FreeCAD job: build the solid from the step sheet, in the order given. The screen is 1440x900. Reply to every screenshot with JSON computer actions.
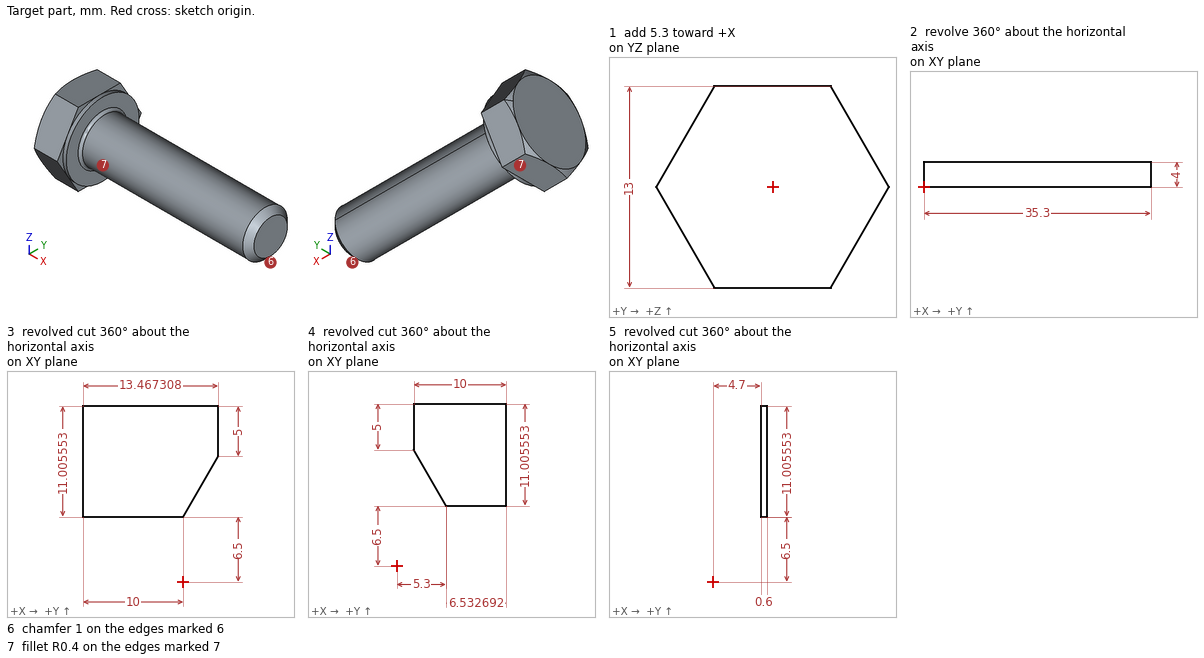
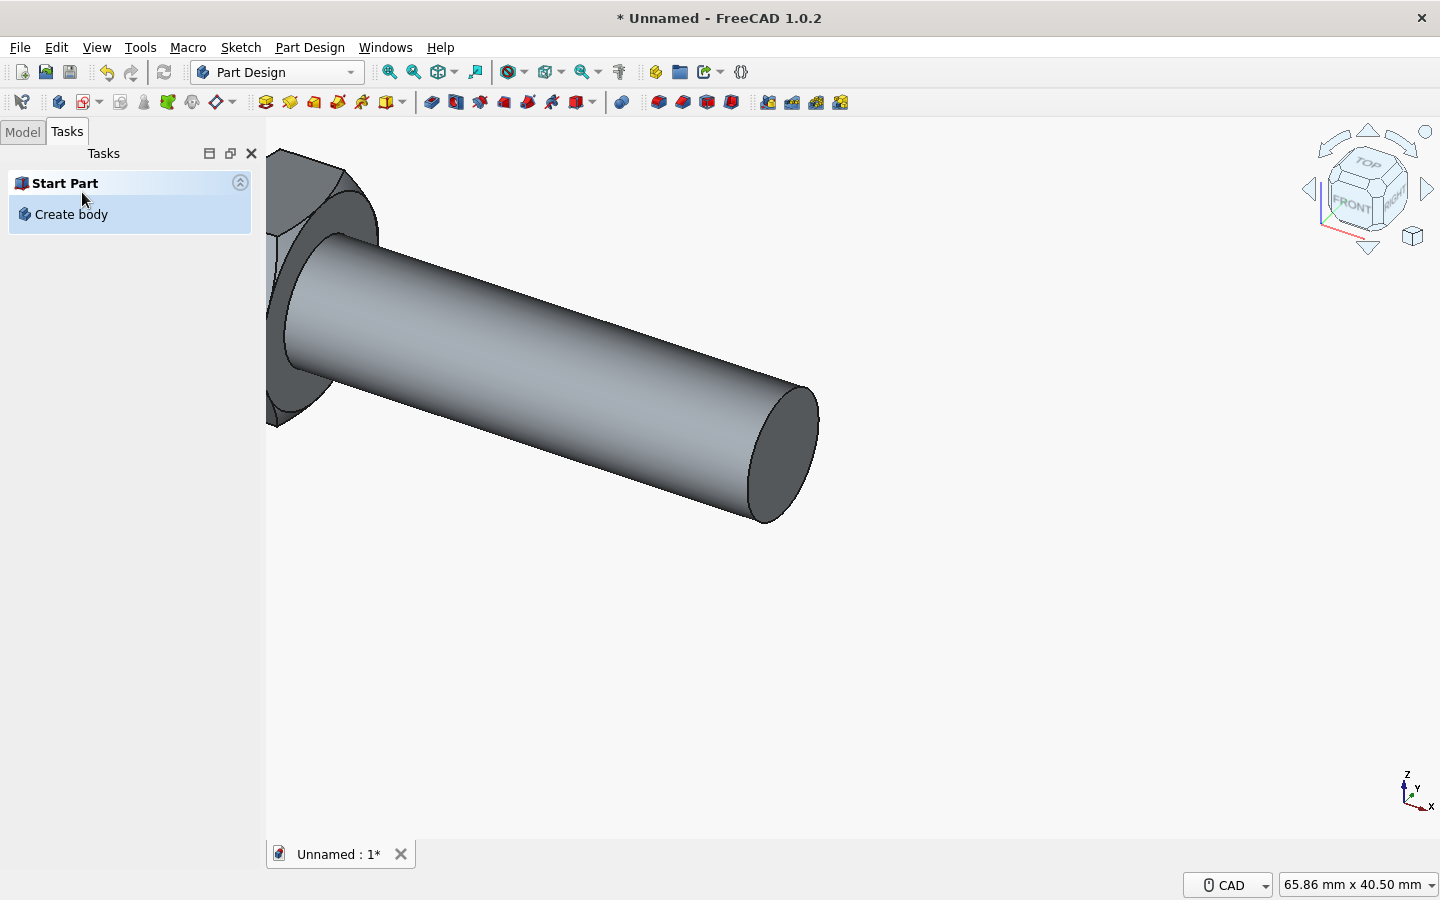
{"action": "key", "text": "v f"}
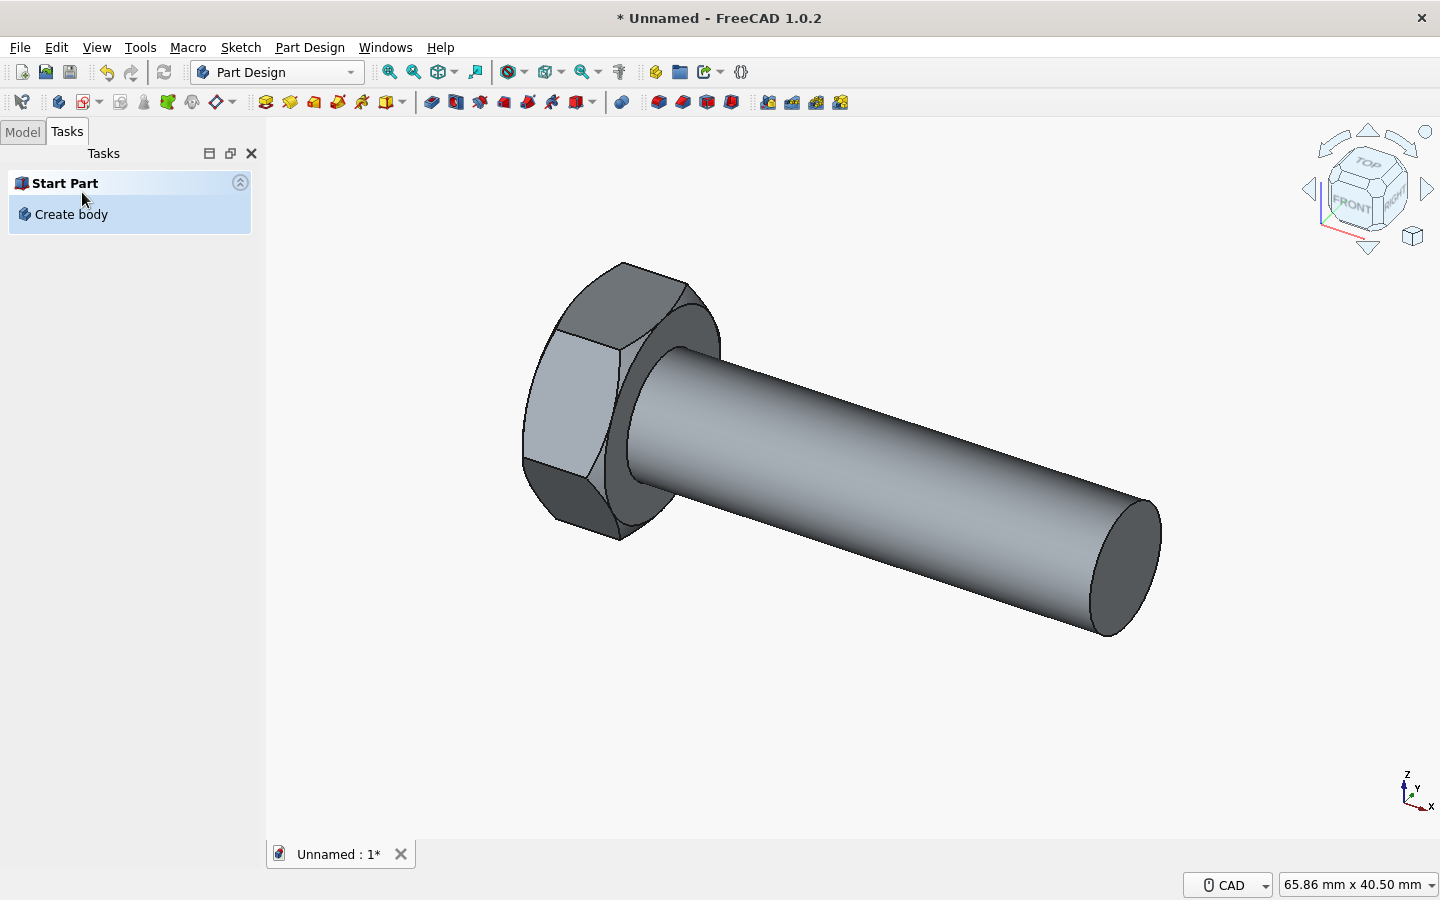
{"action": "left_click", "coordinate": [84, 102]}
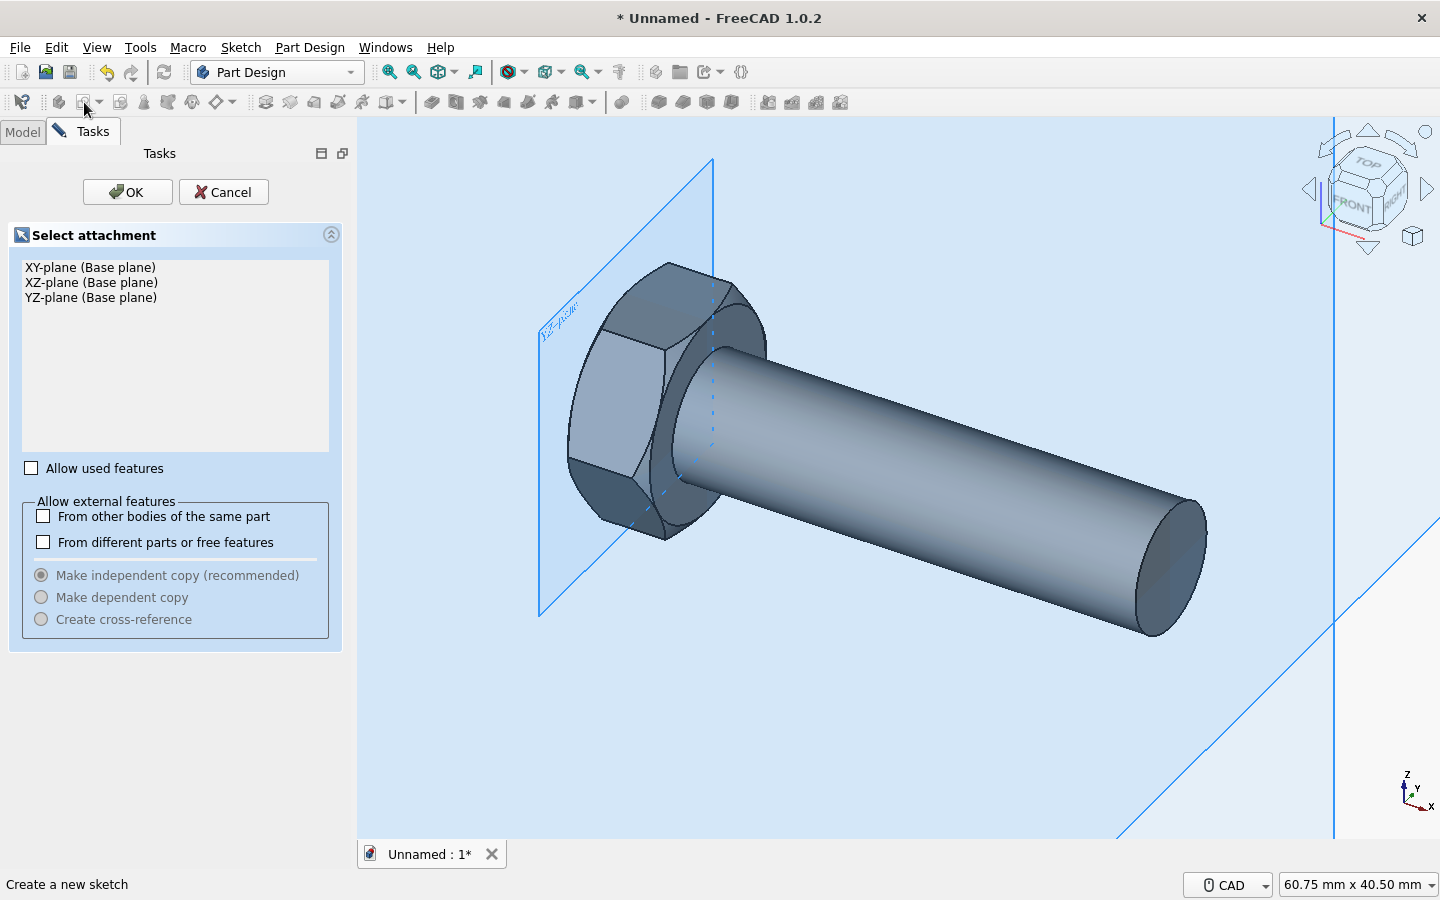
{"action": "left_click", "coordinate": [82, 268]}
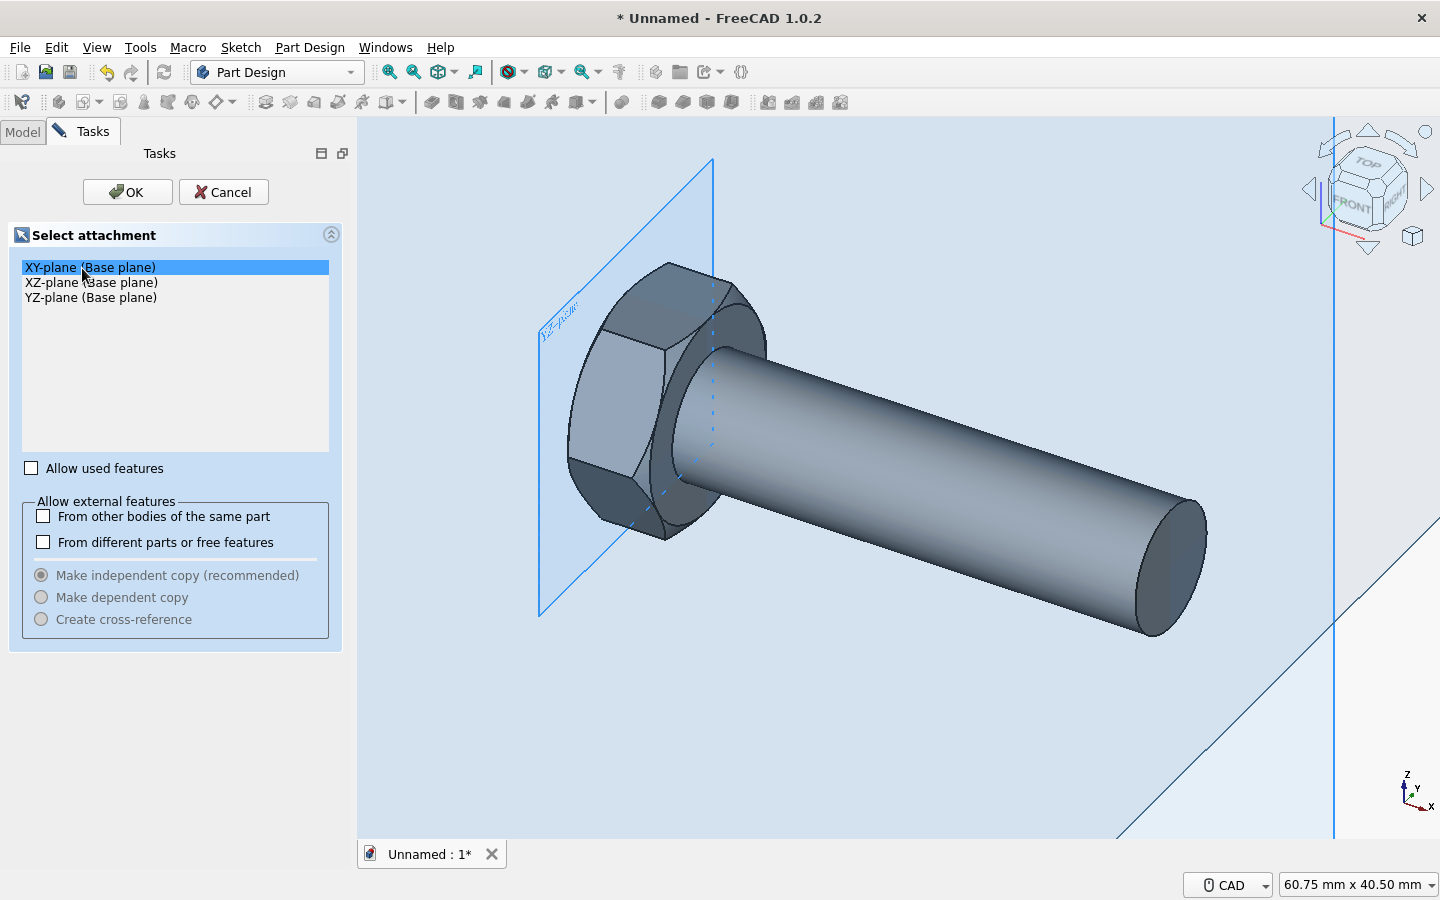
{"action": "left_click", "coordinate": [128, 192]}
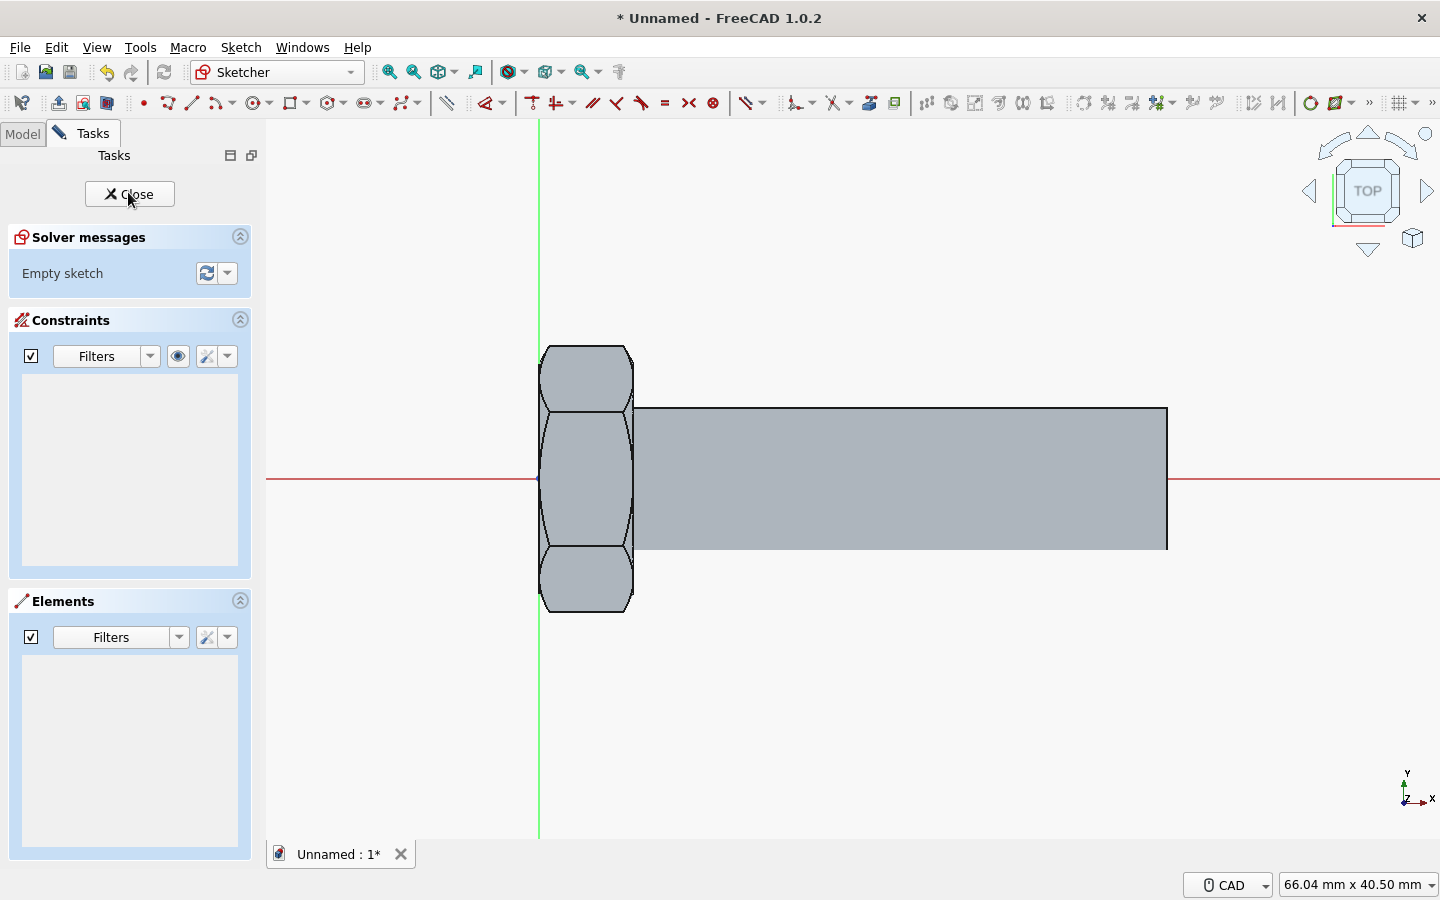
{"action": "key", "text": "q s"}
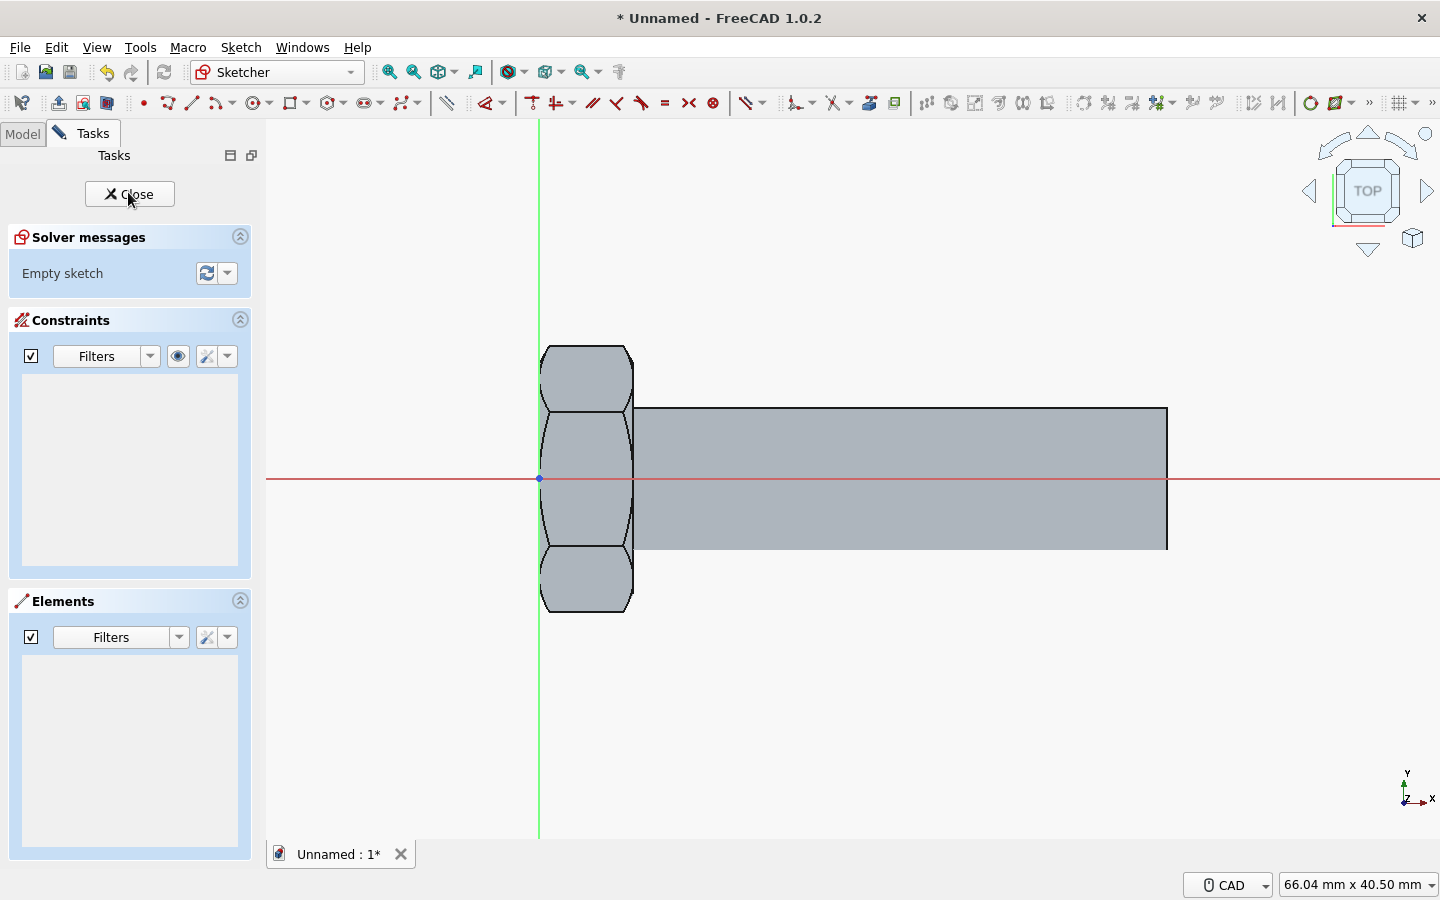
{"action": "scroll", "coordinate": [294, 147], "scroll_direction": "up", "scroll_amount": 2}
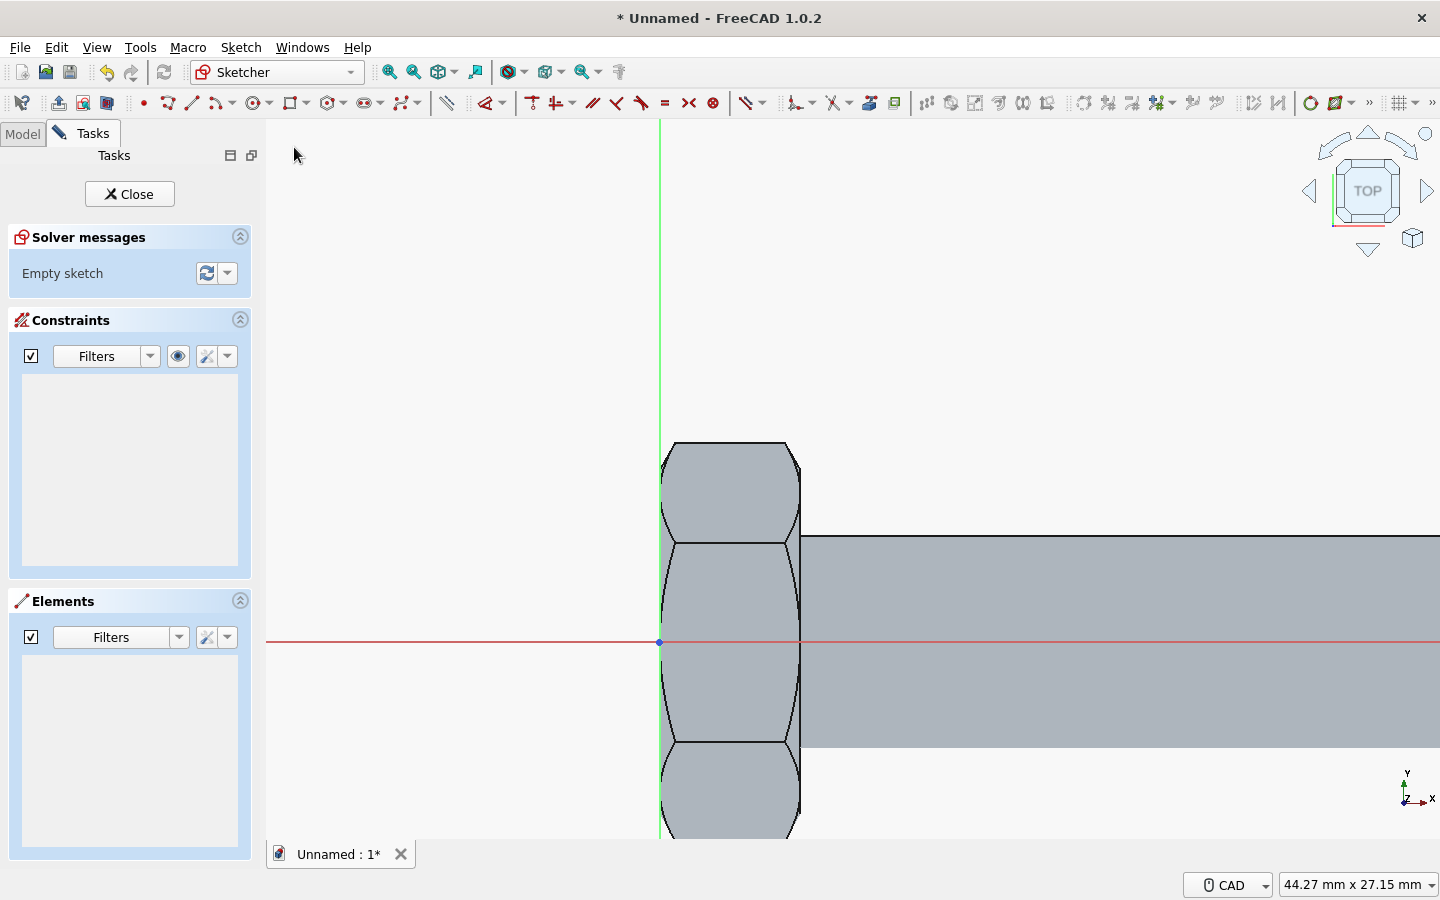
{"action": "key", "text": "g r"}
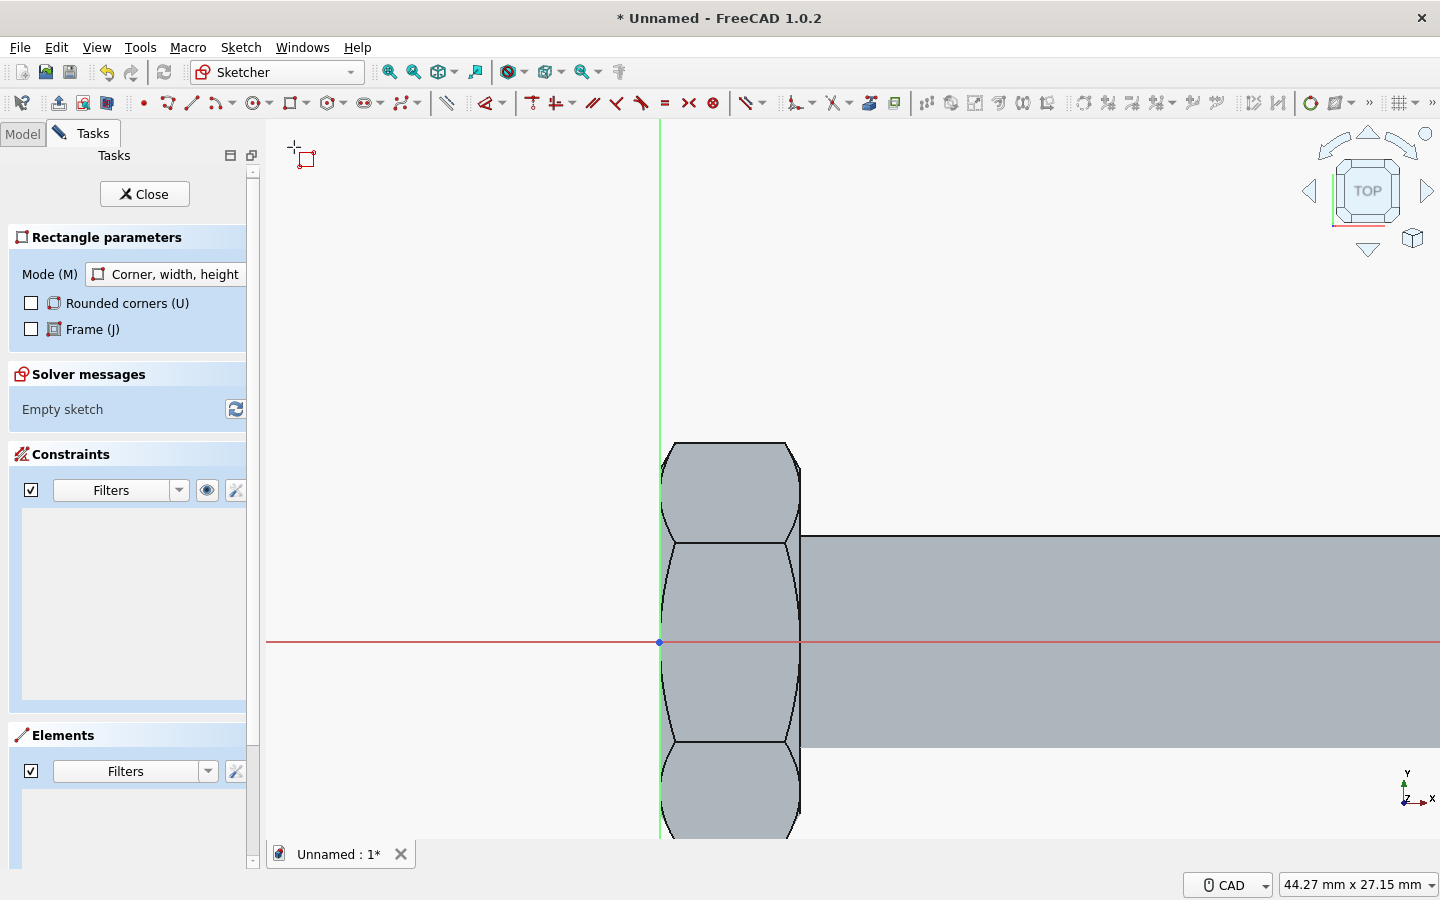
{"action": "left_click", "coordinate": [784, 178]}
{"action": "mouse_move", "coordinate": [800, 470]}